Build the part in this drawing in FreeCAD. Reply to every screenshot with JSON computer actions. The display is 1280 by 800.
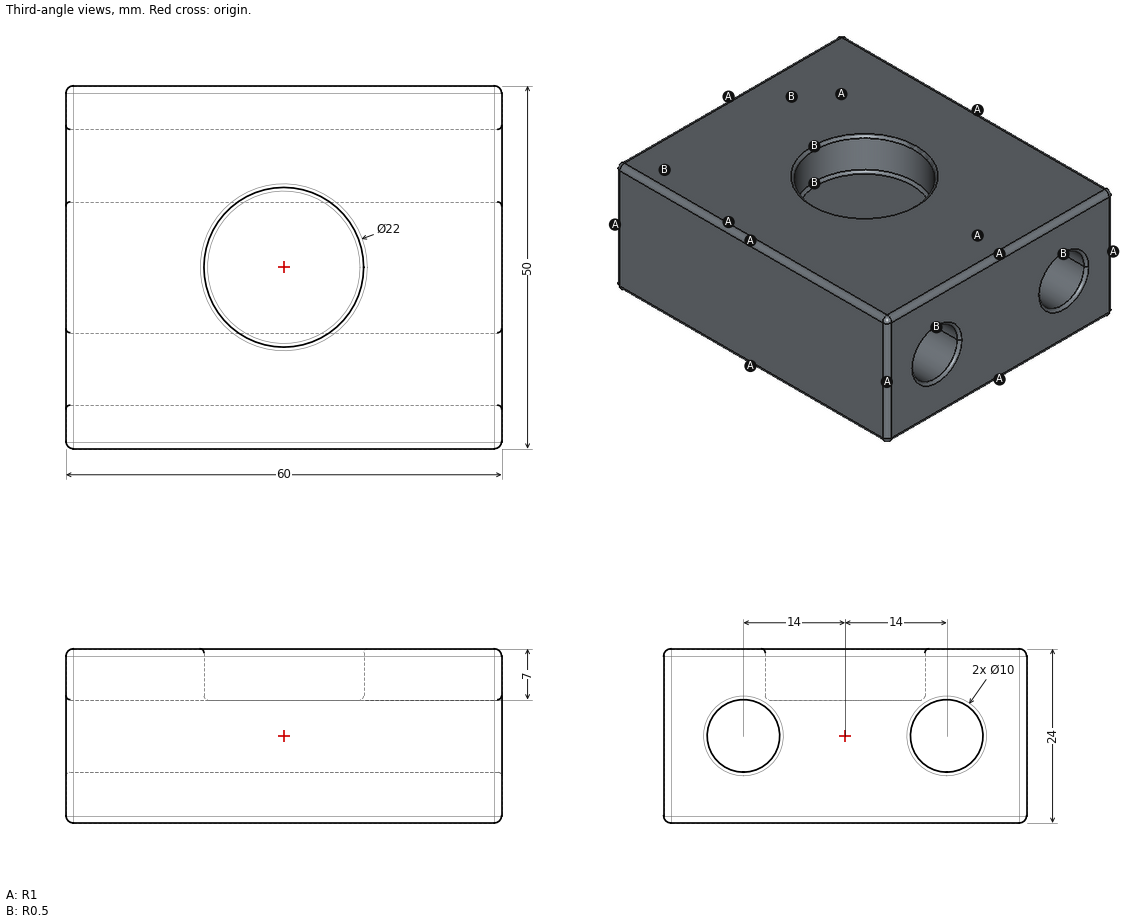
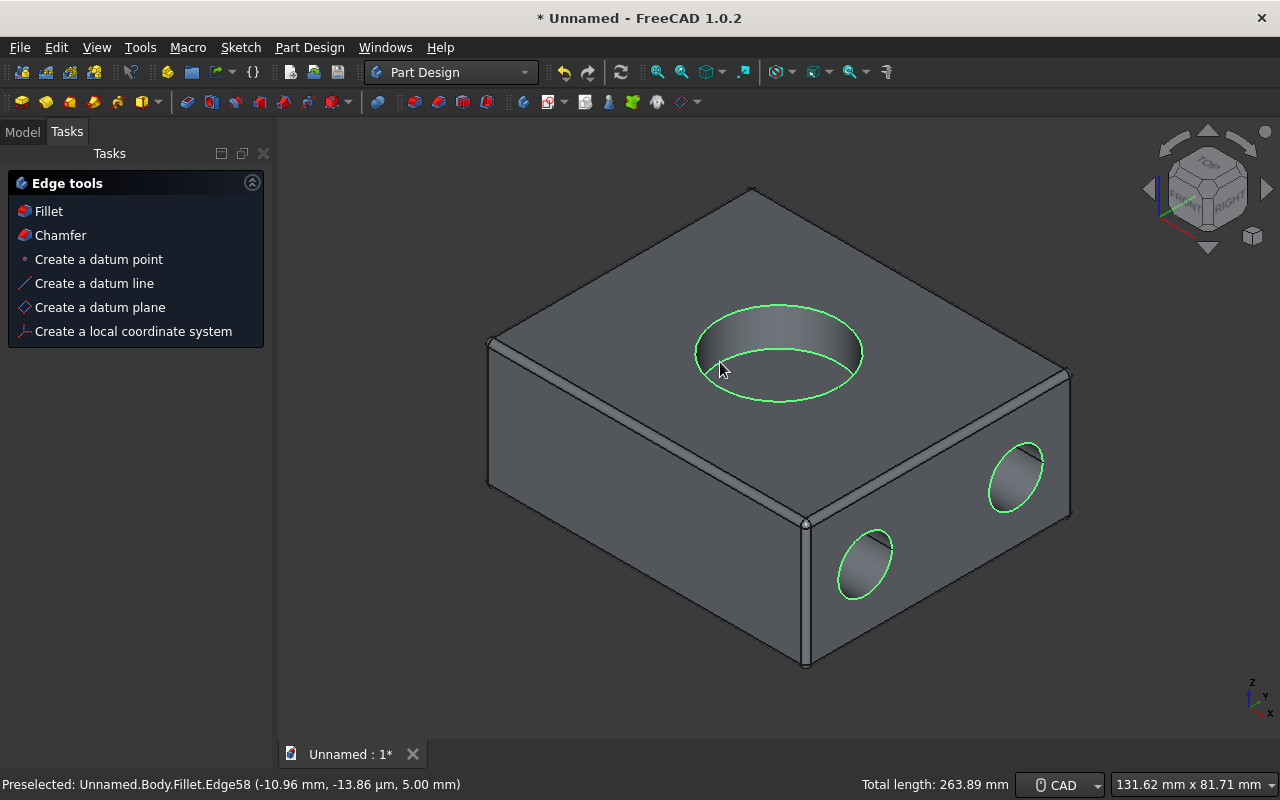
{"action": "left_click", "coordinate": [416, 102]}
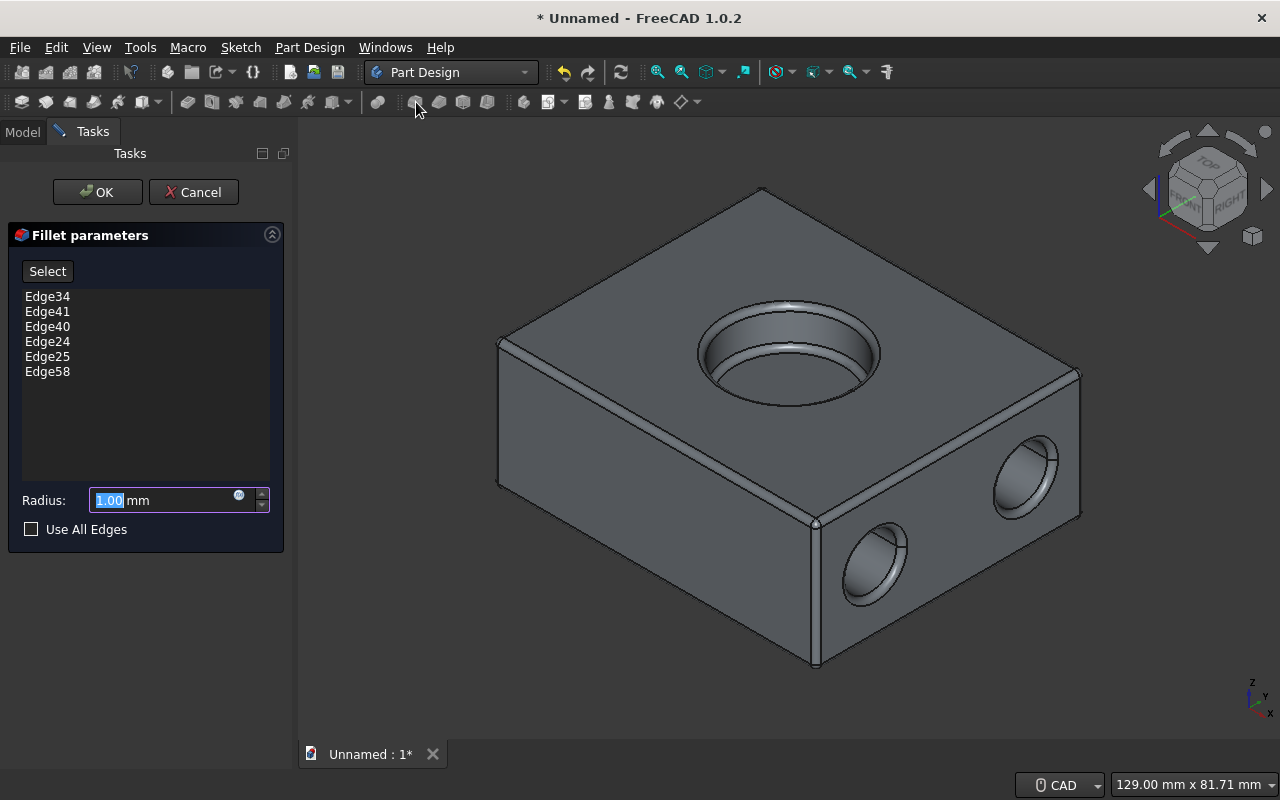
{"action": "type", "text": "0.5"}
{"action": "key", "text": "Tab"}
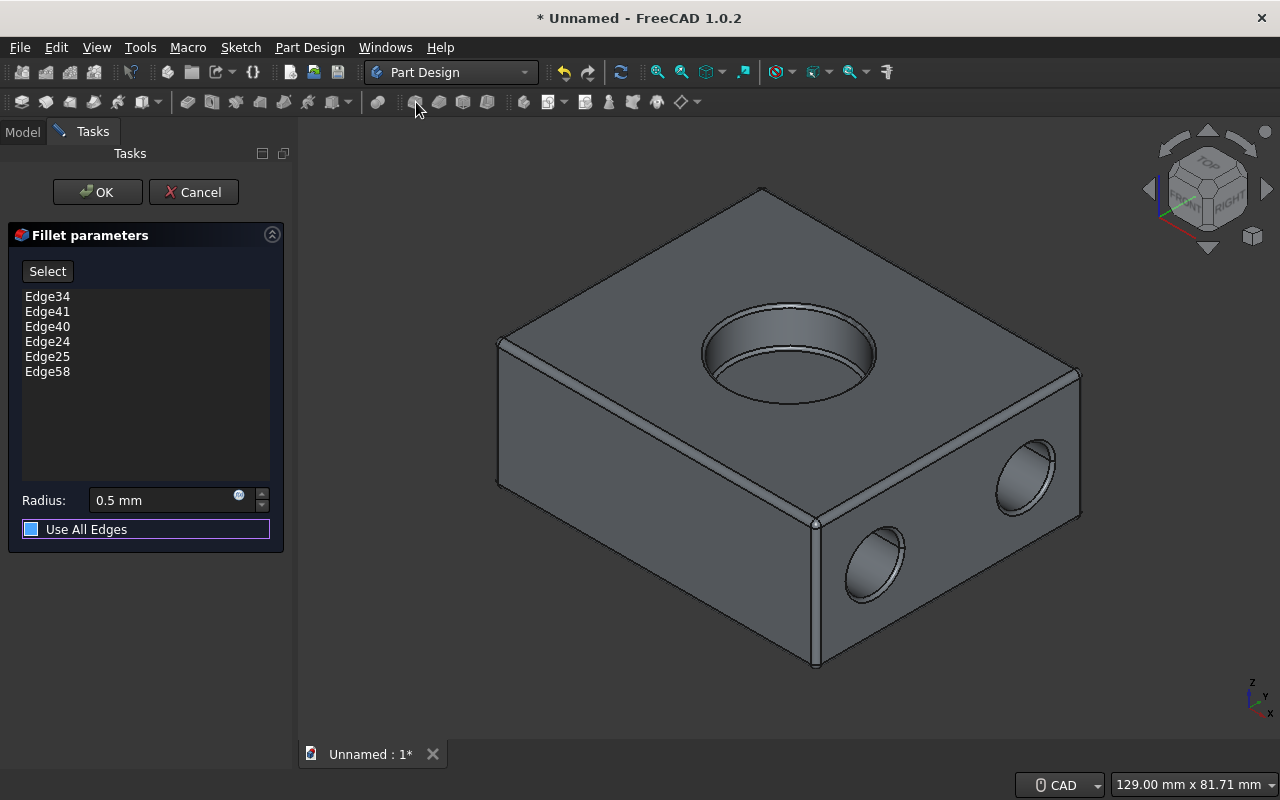
{"action": "left_click", "coordinate": [98, 192]}